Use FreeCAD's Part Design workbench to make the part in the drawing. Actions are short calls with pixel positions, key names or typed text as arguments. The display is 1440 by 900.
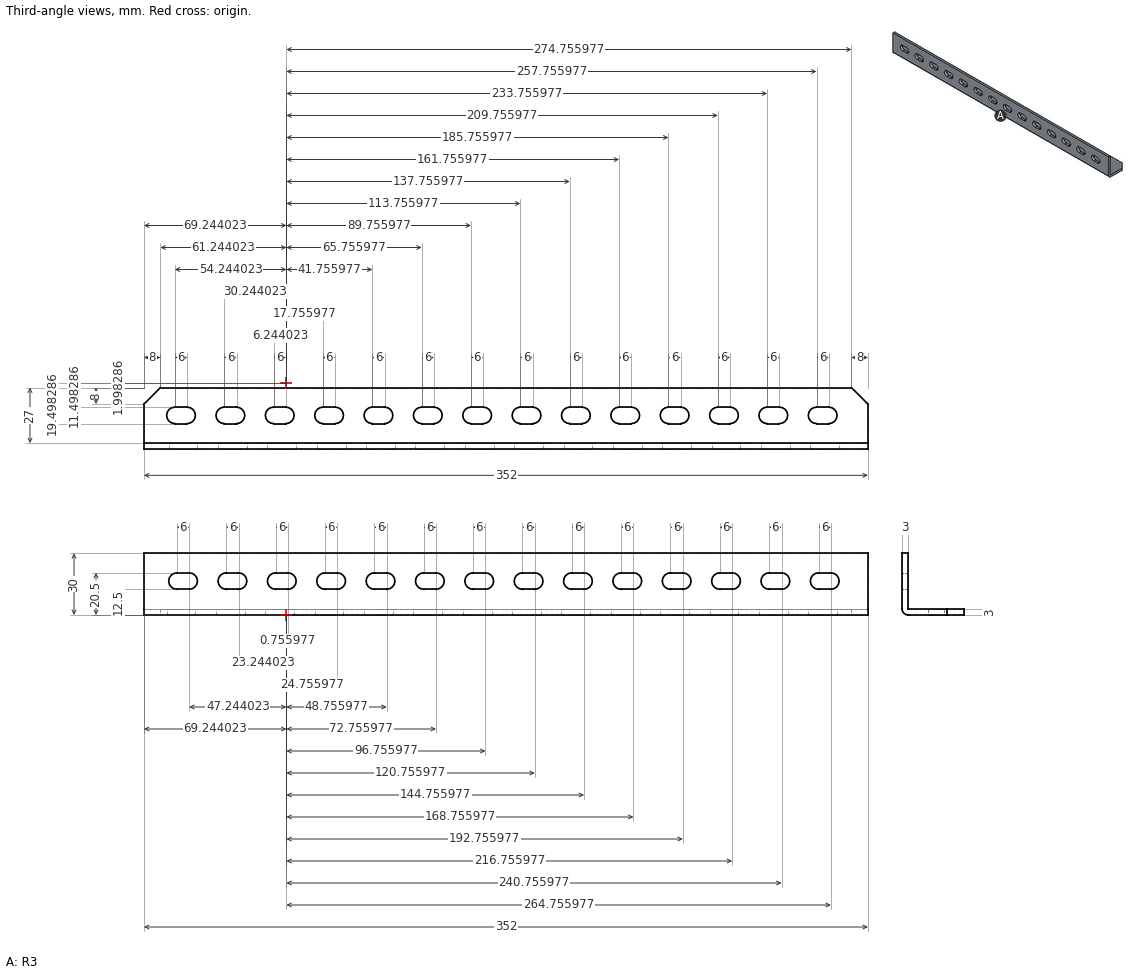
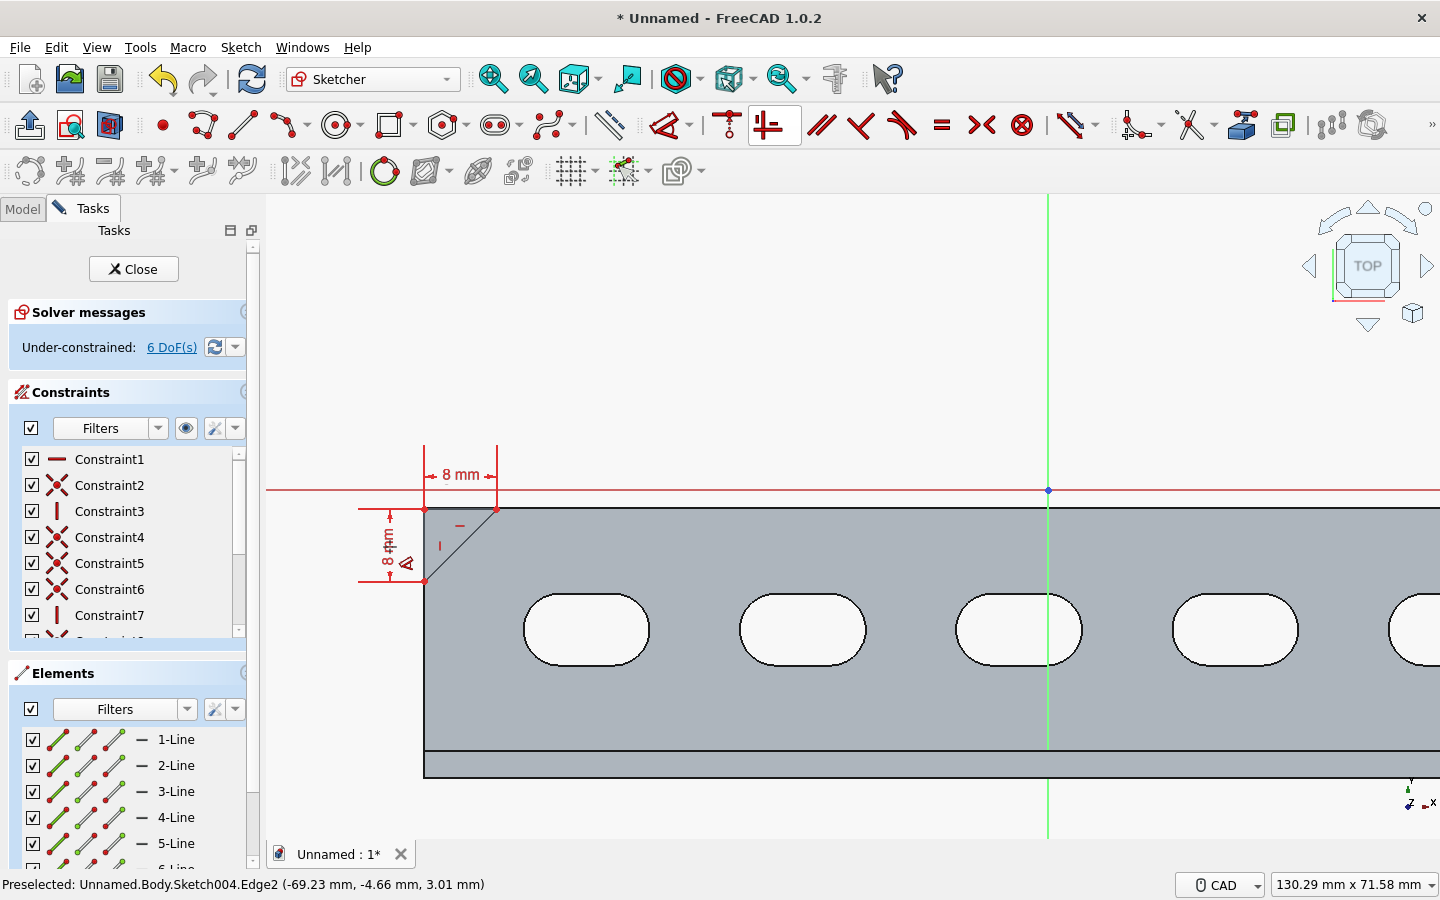
scroll(474, 512, down, 8)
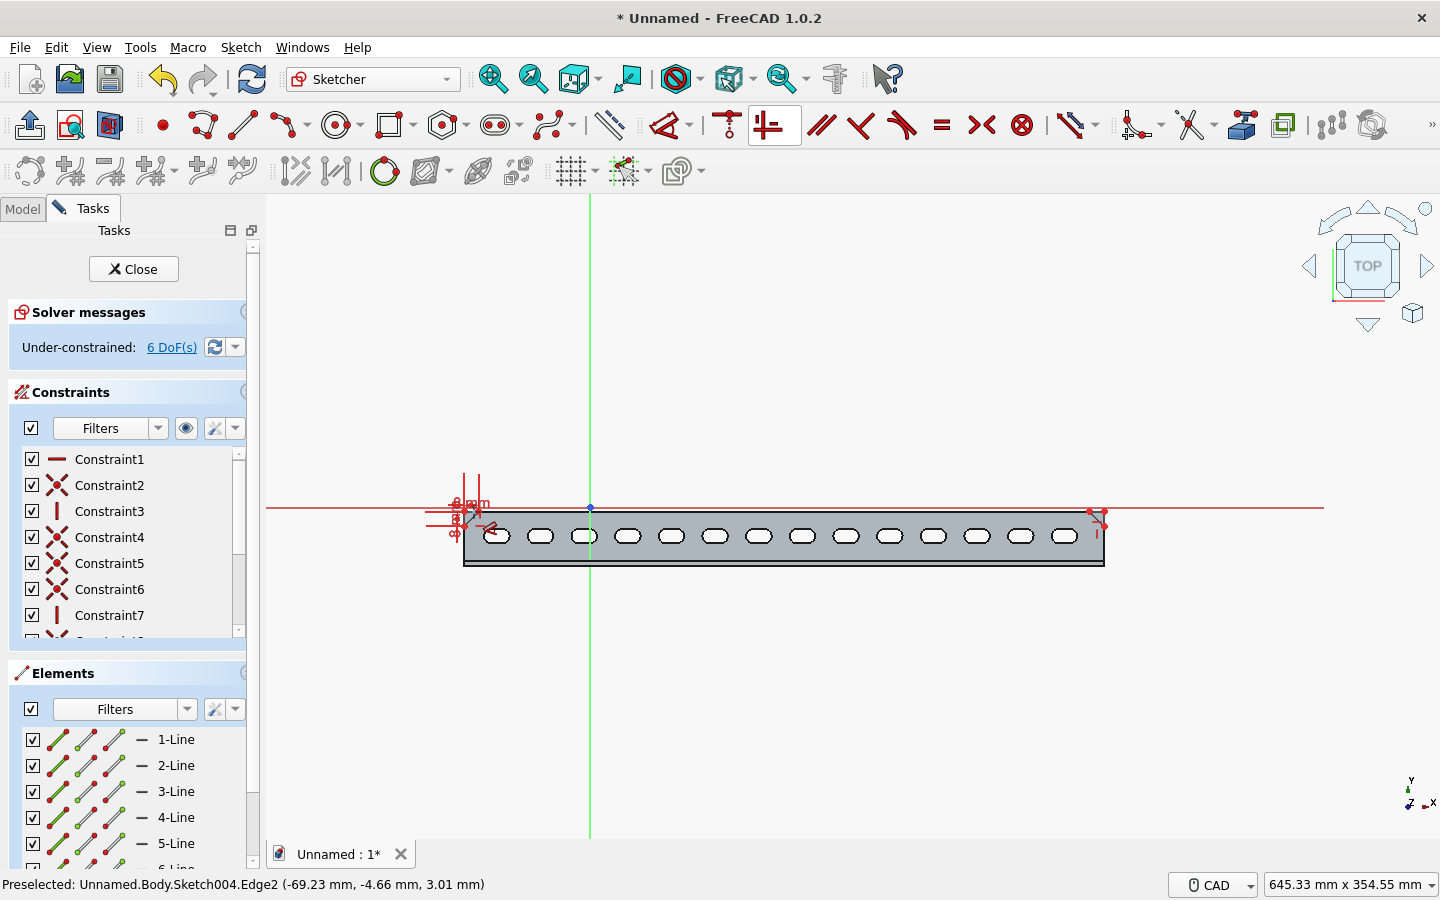
scroll(1104, 522, up, 8)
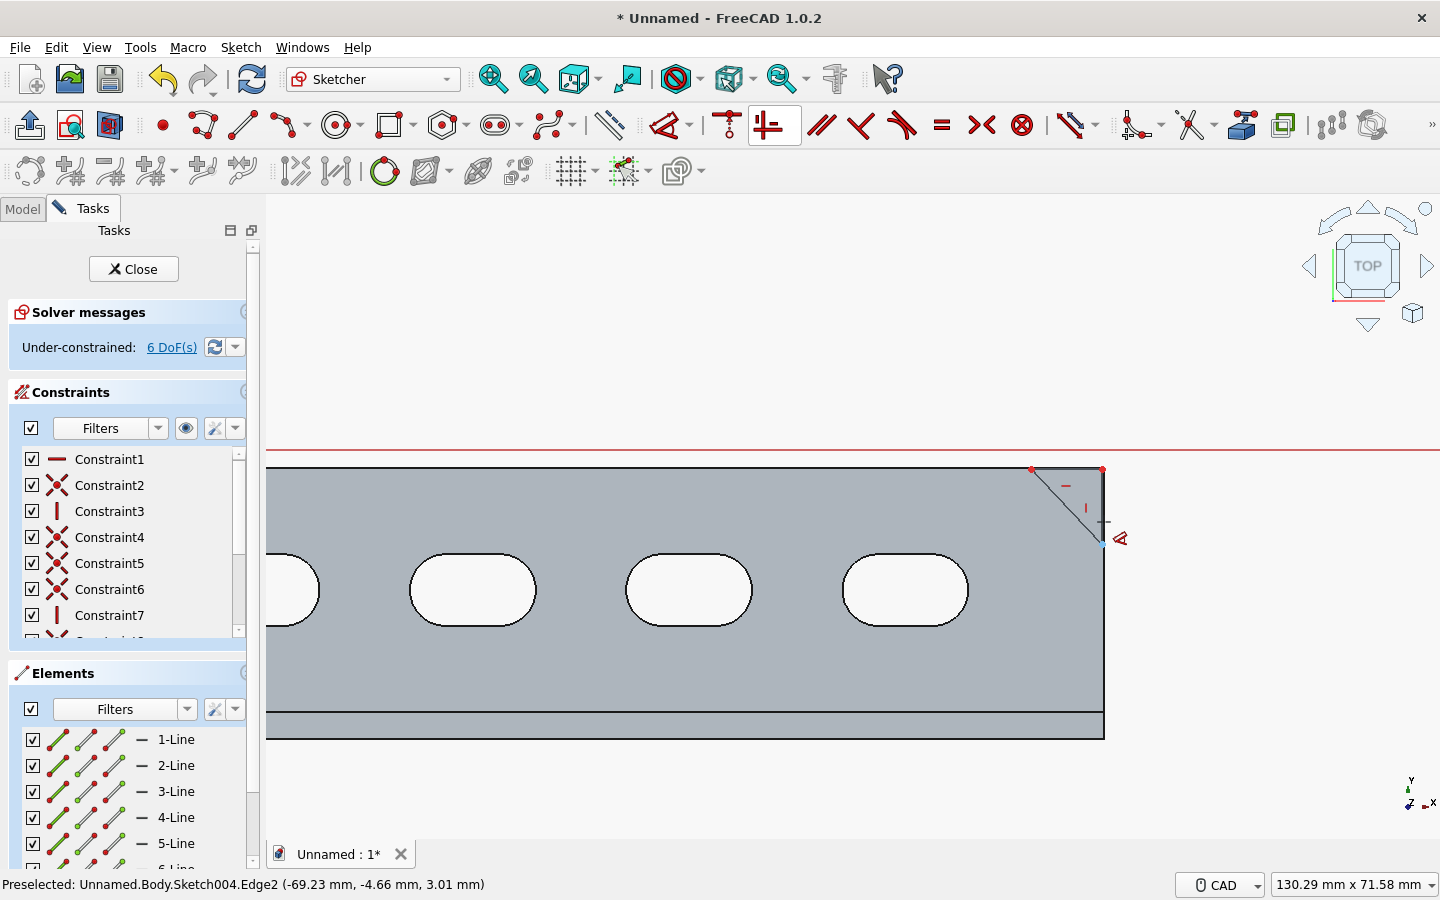
click(1102, 522)
click(1136, 507)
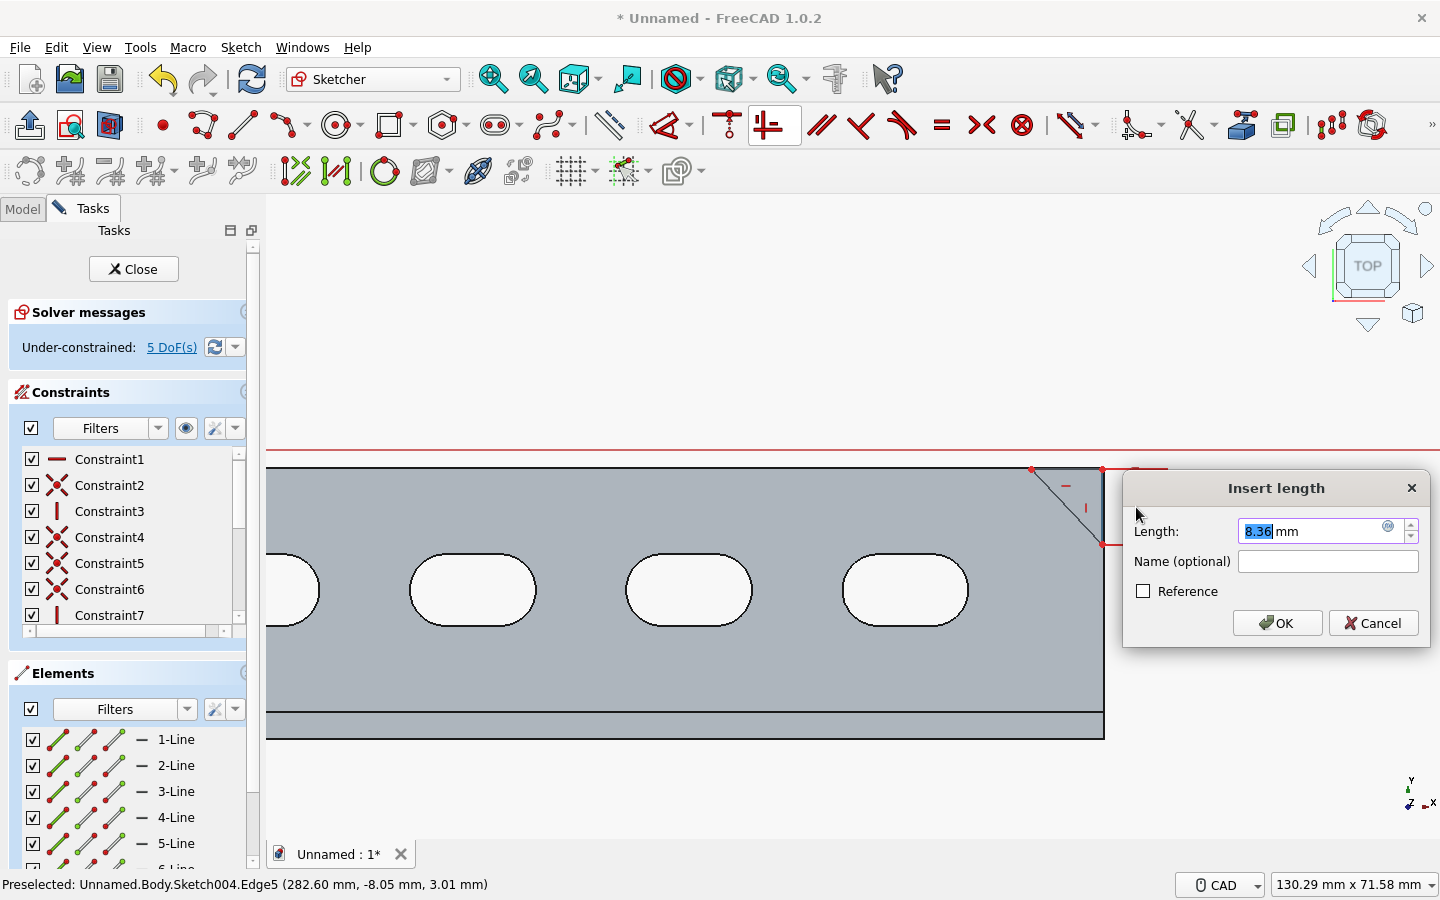
text(8)
key(Return)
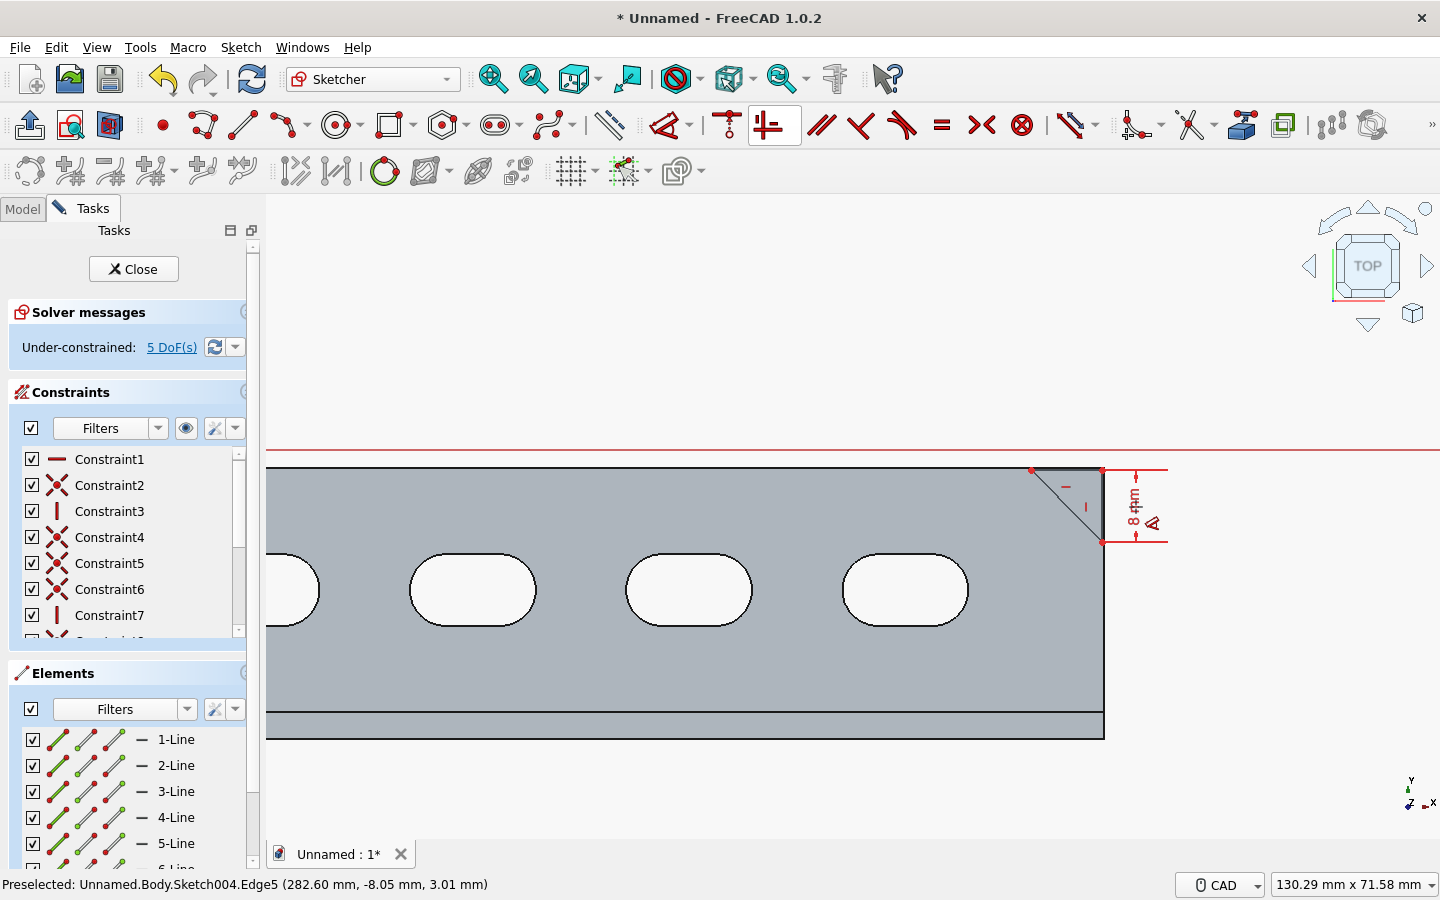
click(1081, 470)
click(1067, 436)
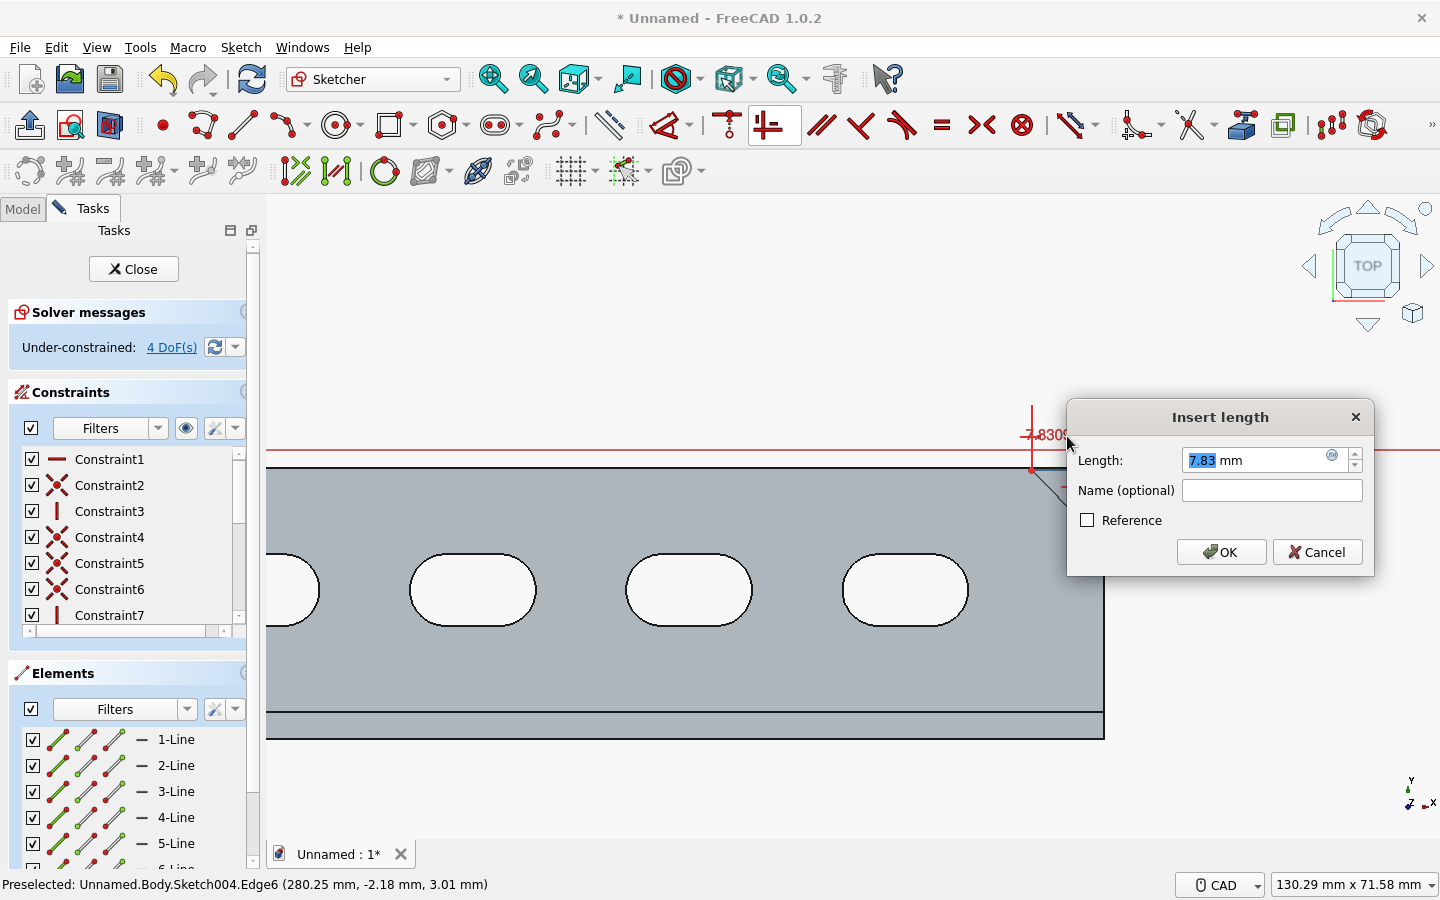
text(8)
key(Return)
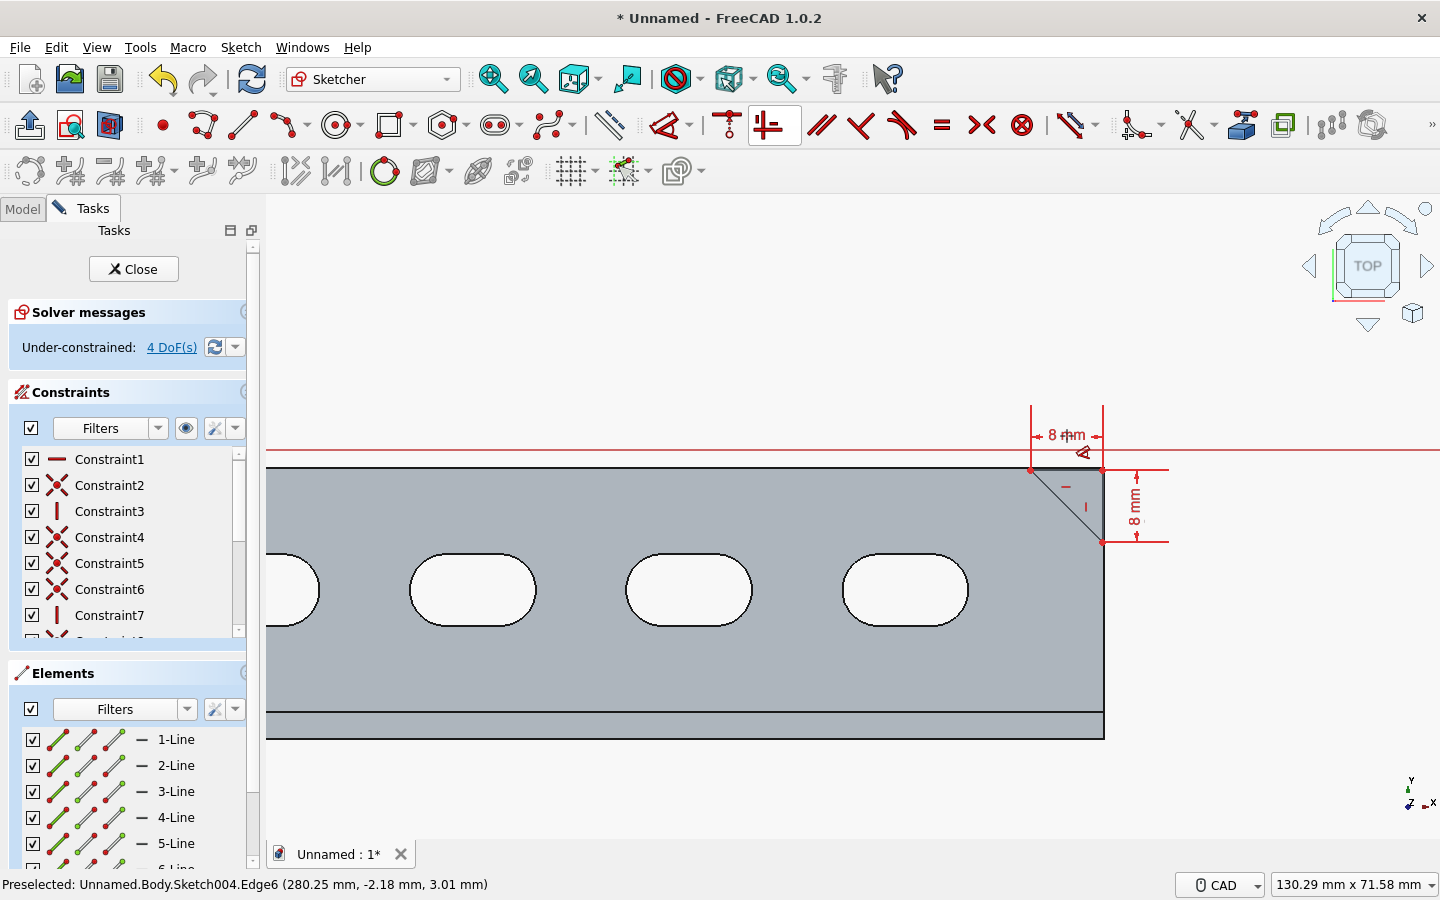
scroll(1105, 522, down, 8)